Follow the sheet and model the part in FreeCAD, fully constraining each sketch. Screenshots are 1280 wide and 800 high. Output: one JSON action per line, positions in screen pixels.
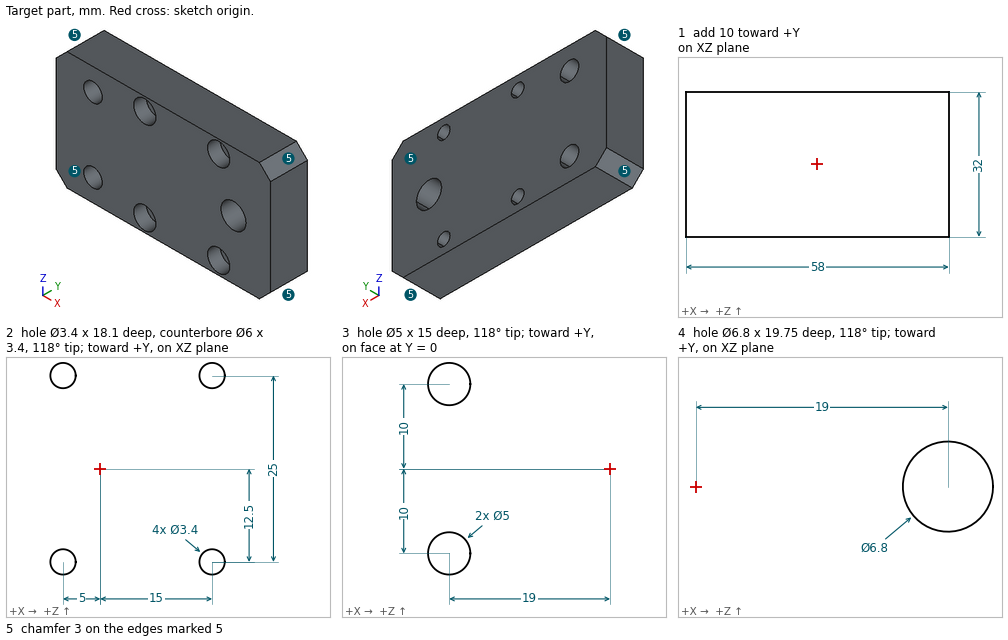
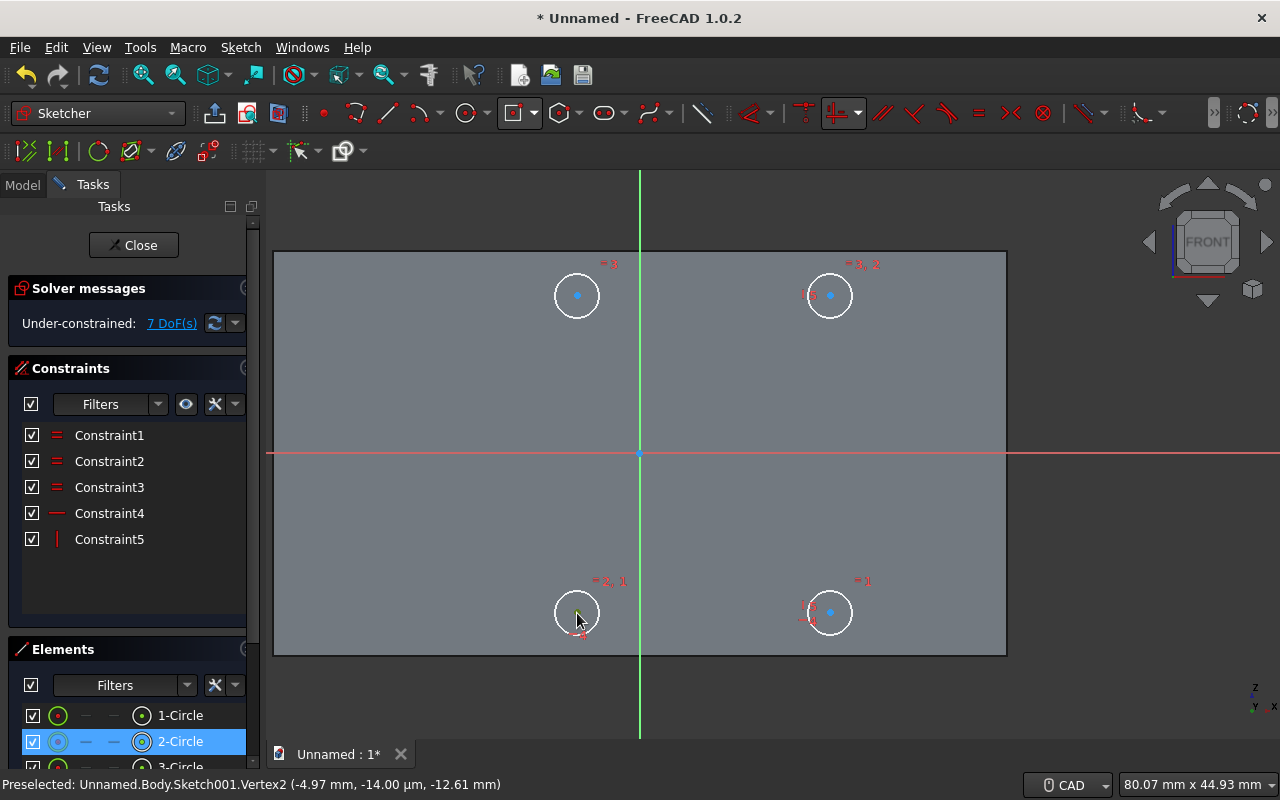
{"action": "left_click", "coordinate": [577, 296]}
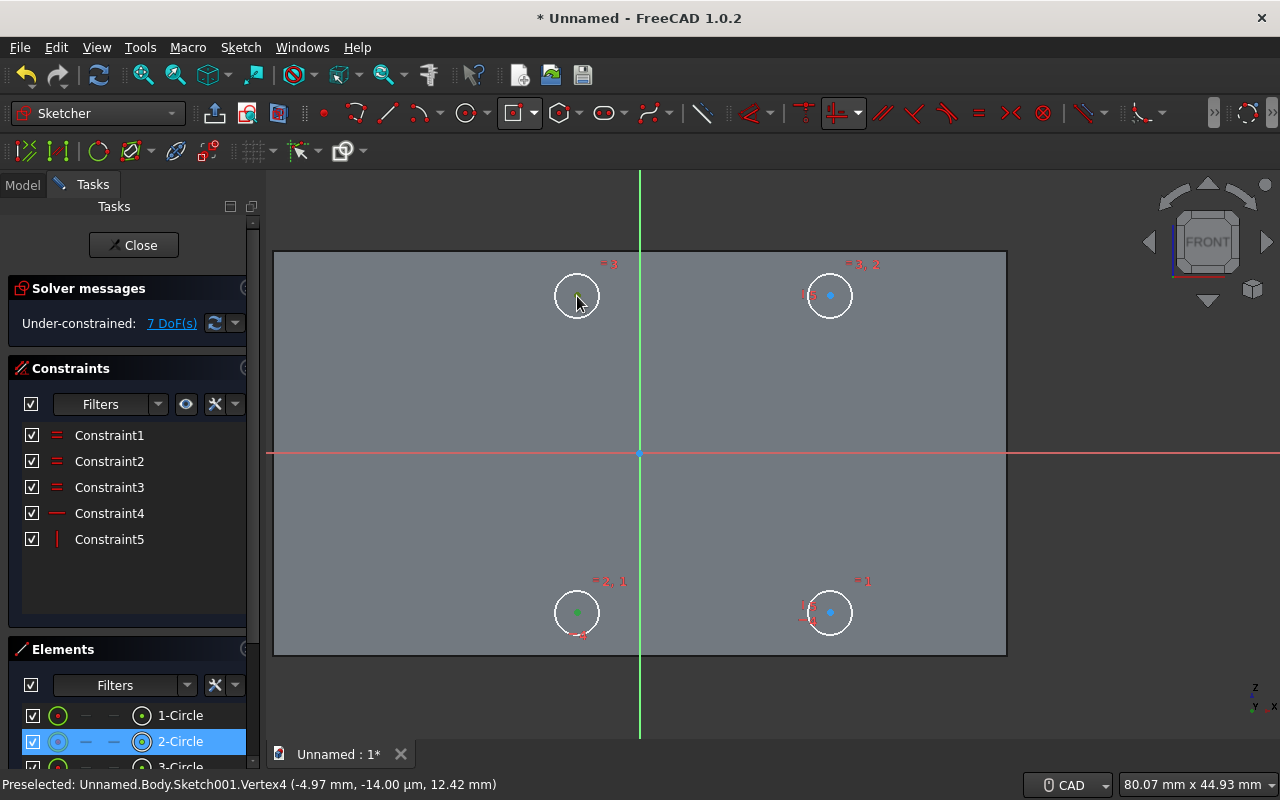
{"action": "left_click", "coordinate": [860, 114]}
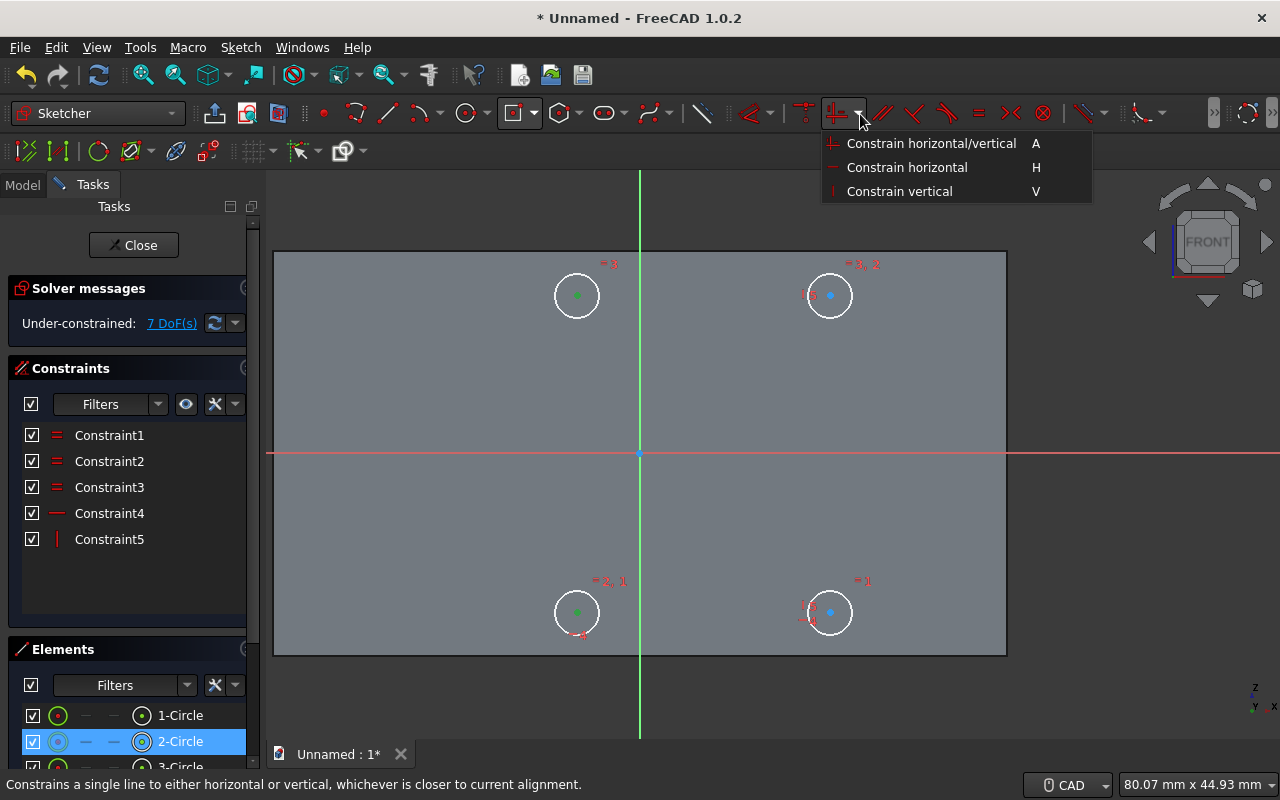
{"action": "left_click", "coordinate": [957, 191]}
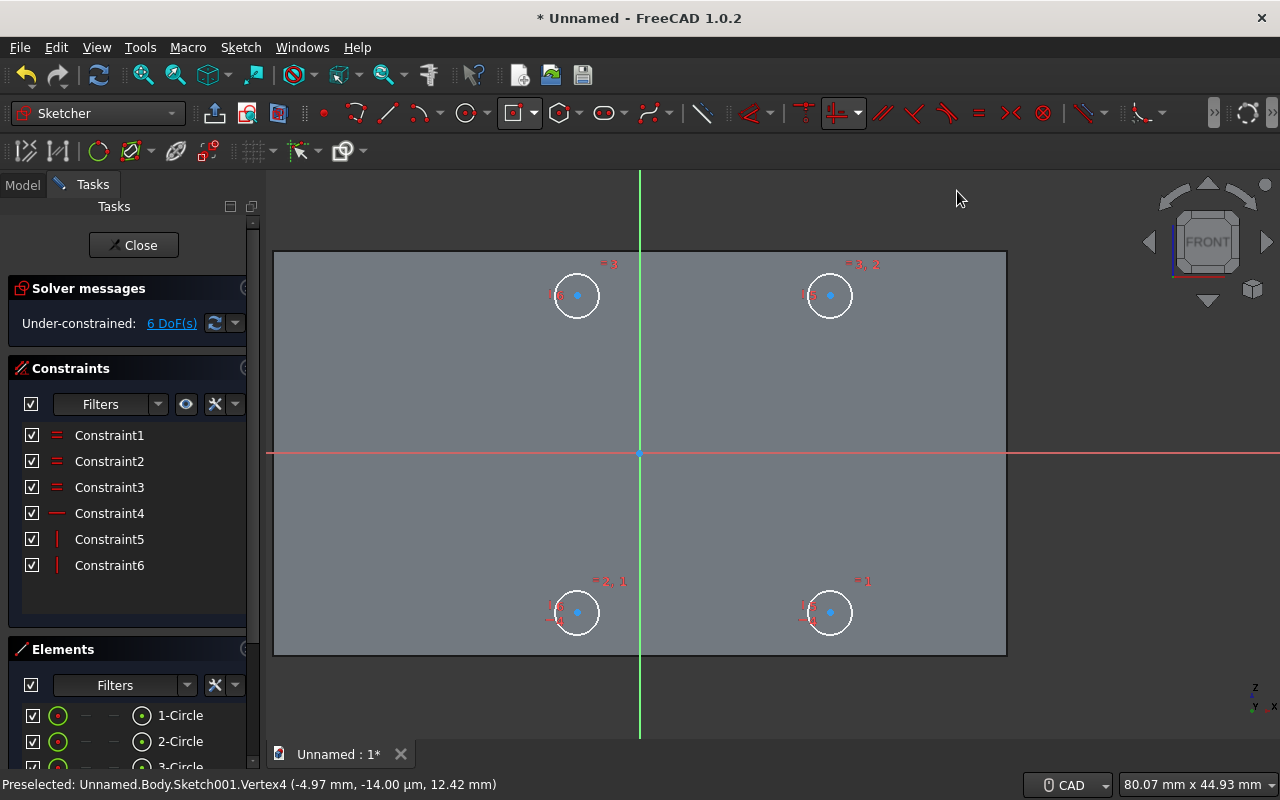
{"action": "left_click", "coordinate": [830, 296]}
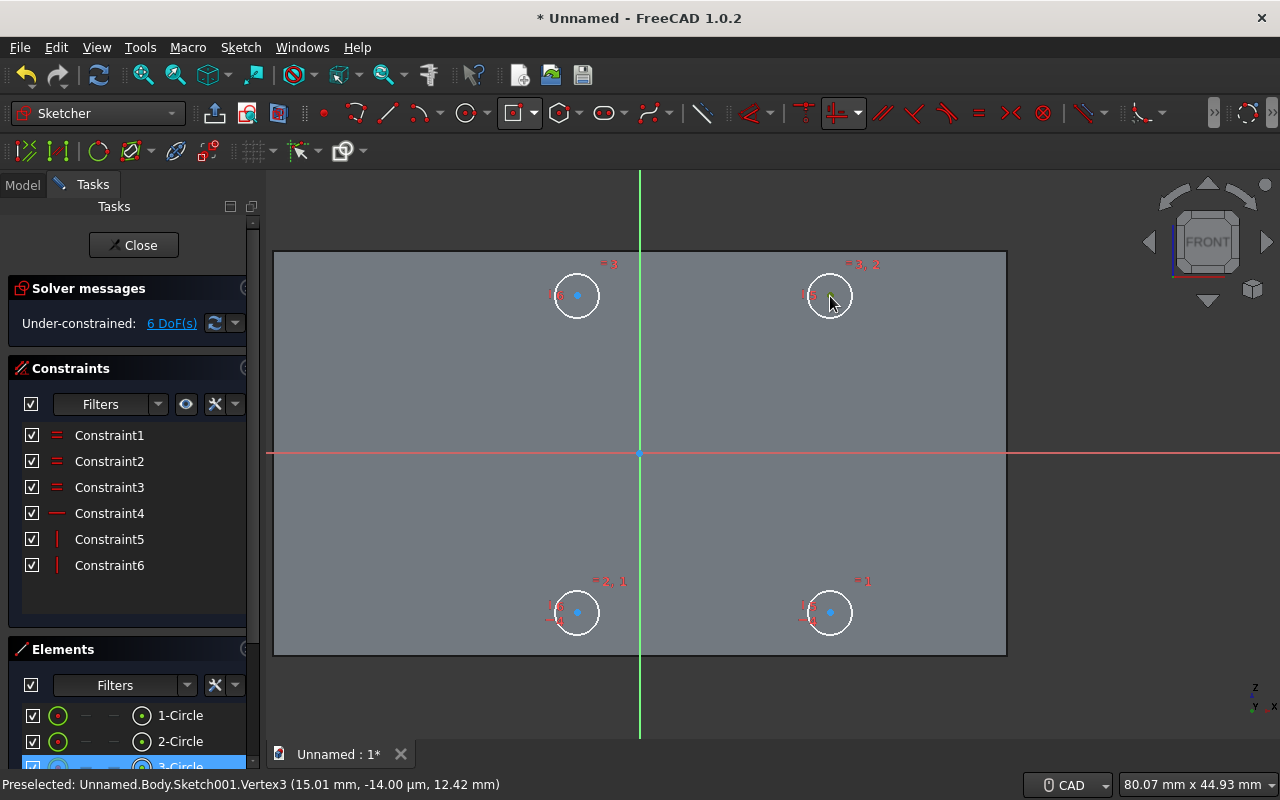
{"action": "left_click", "coordinate": [577, 296]}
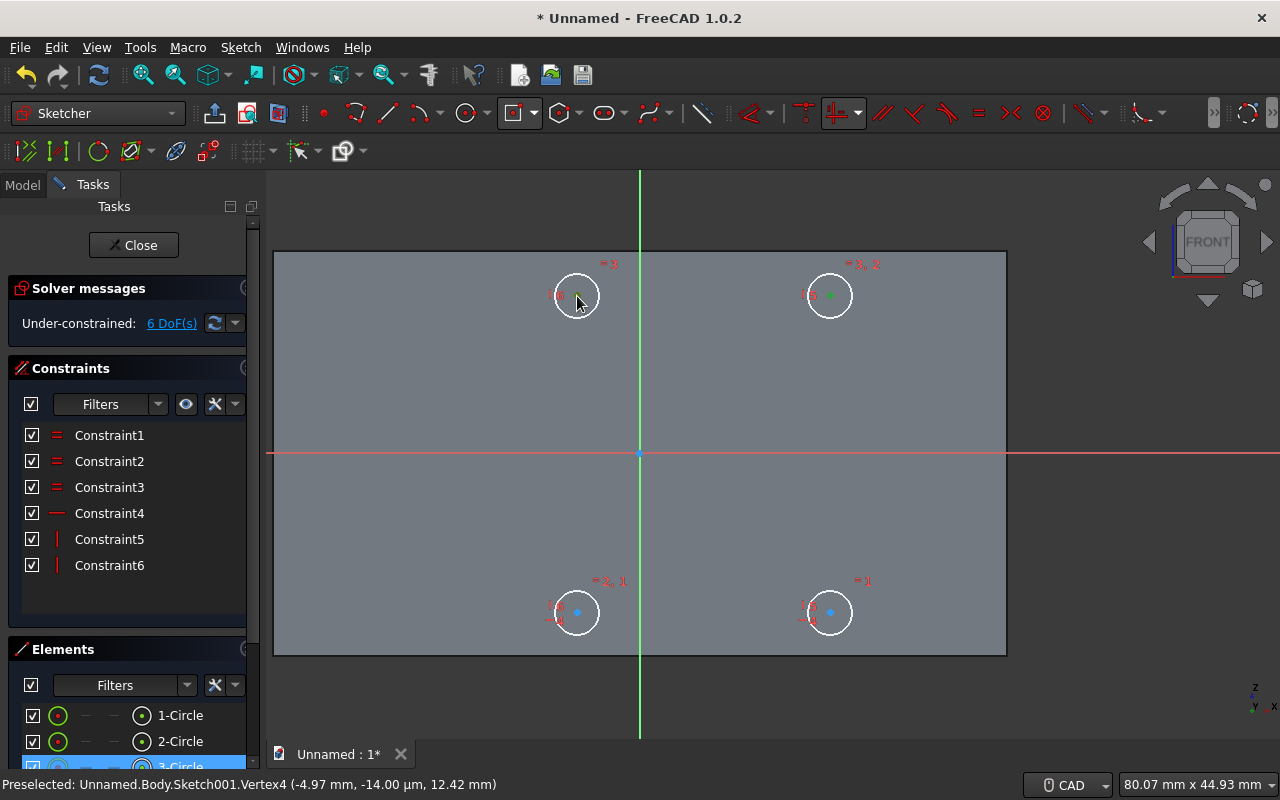
{"action": "left_click", "coordinate": [860, 114]}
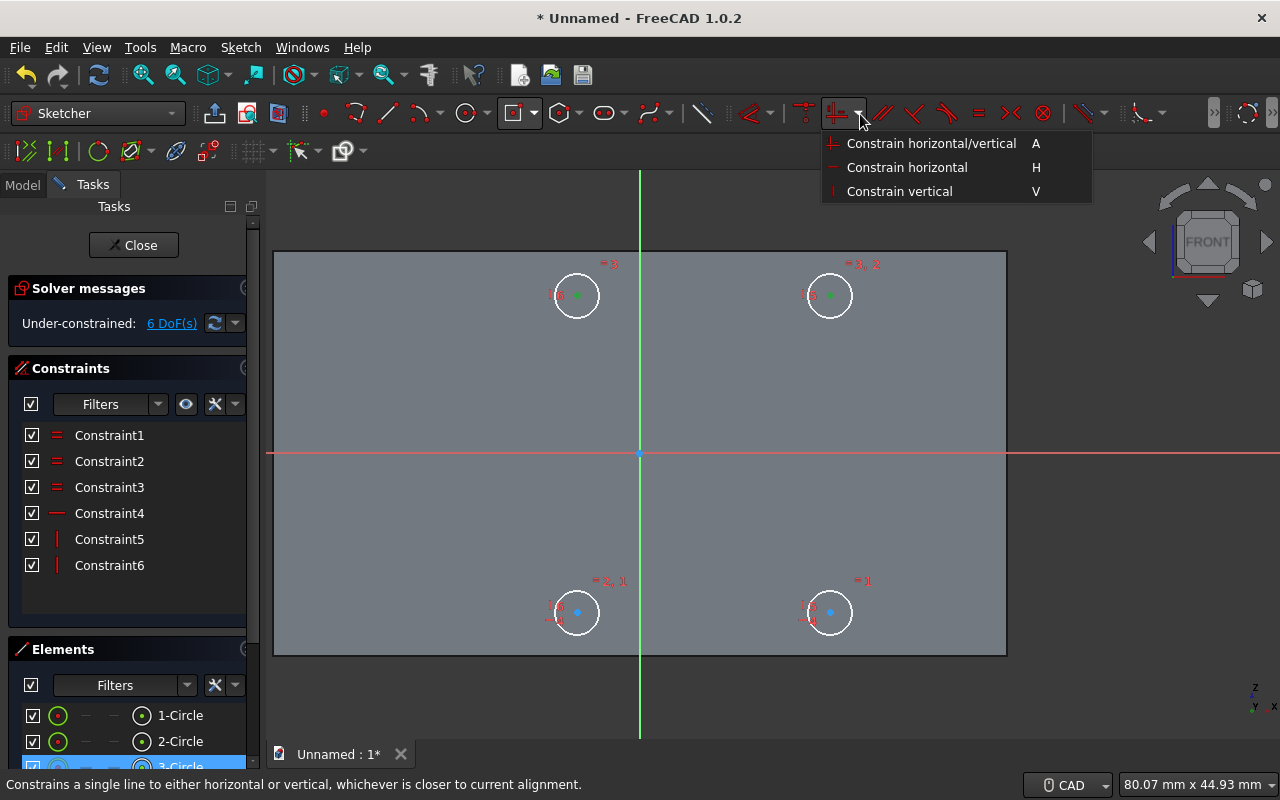
{"action": "left_click", "coordinate": [957, 167]}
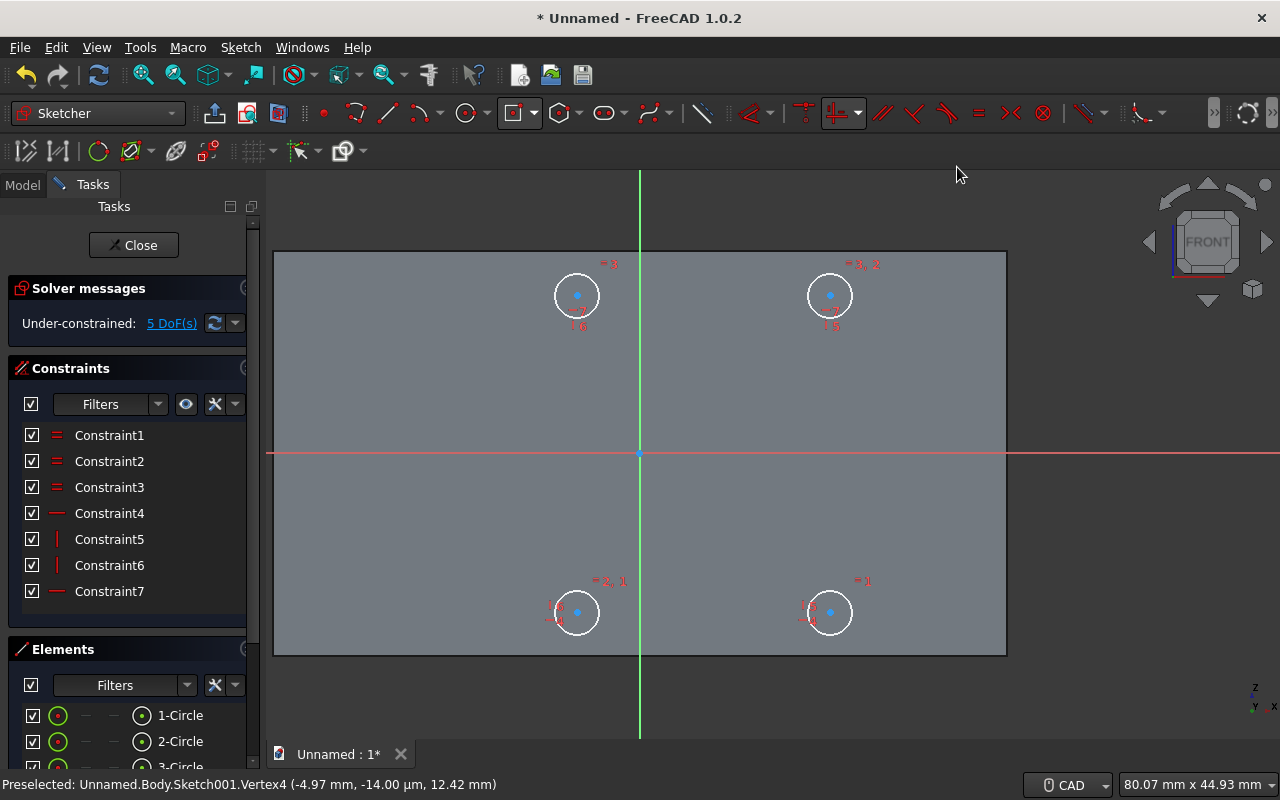
{"action": "left_click", "coordinate": [750, 114]}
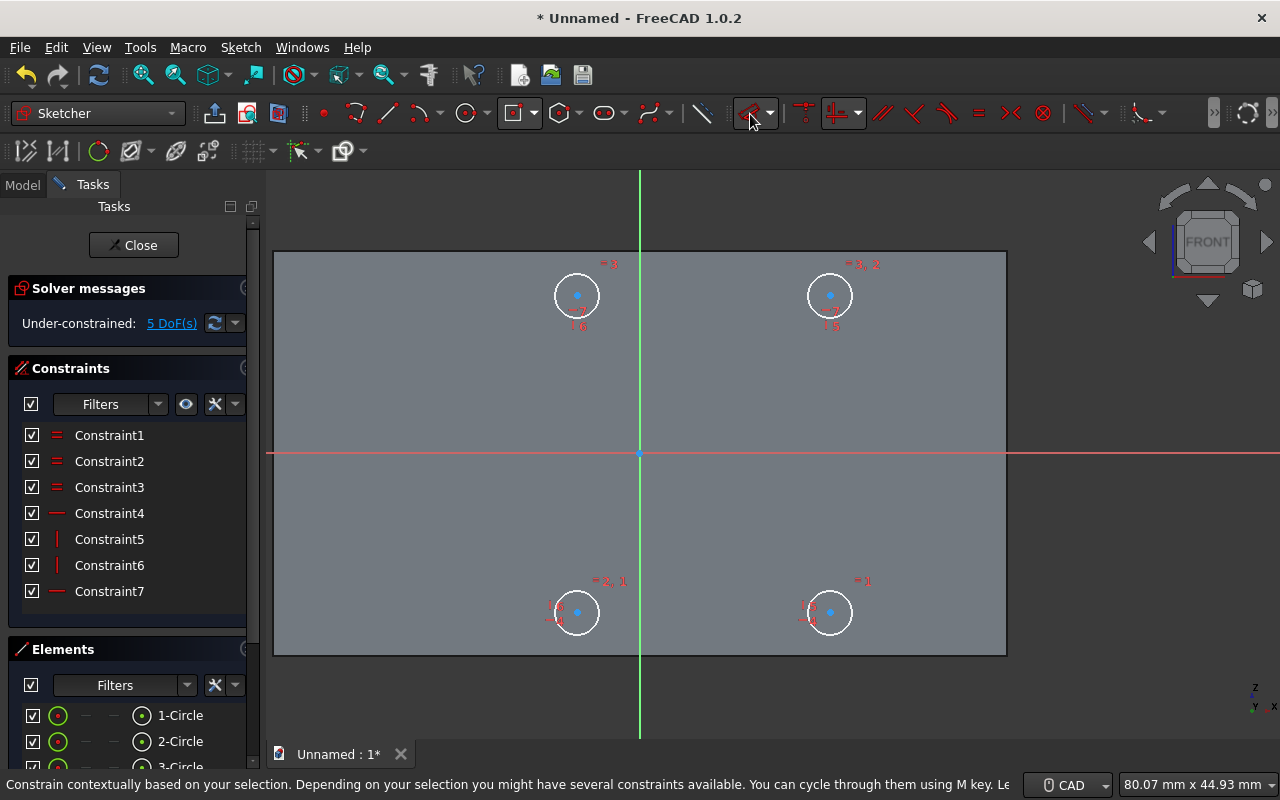
{"action": "left_click", "coordinate": [845, 597]}
{"action": "left_click", "coordinate": [867, 574]}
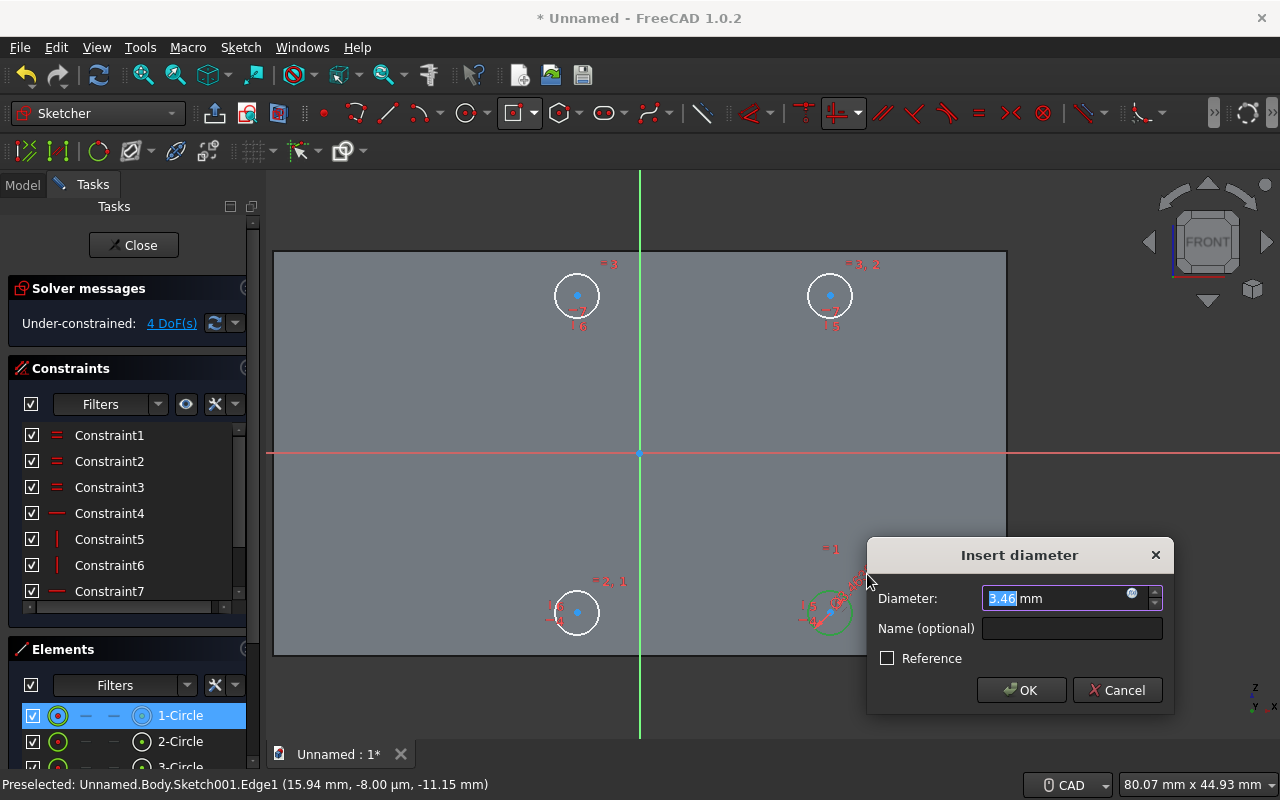
{"action": "type", "text": "3.4"}
{"action": "key", "text": "Return"}